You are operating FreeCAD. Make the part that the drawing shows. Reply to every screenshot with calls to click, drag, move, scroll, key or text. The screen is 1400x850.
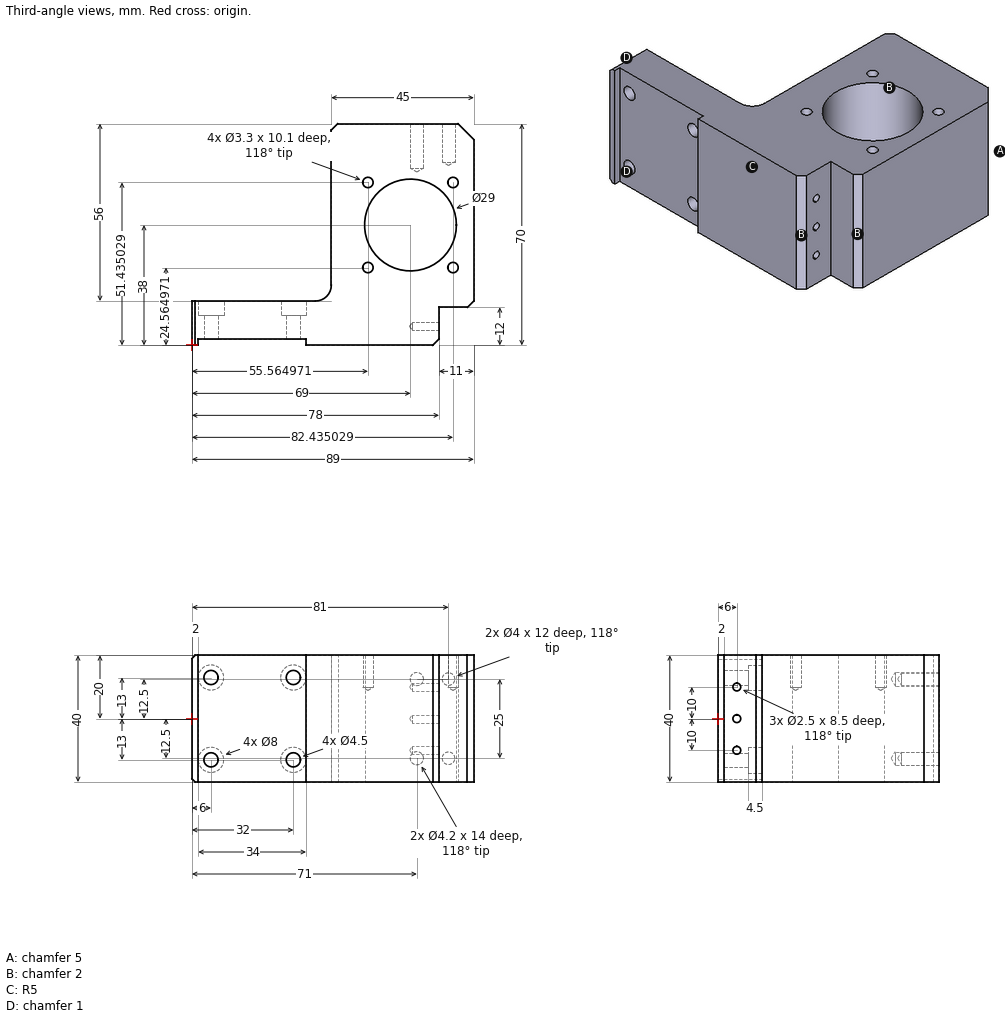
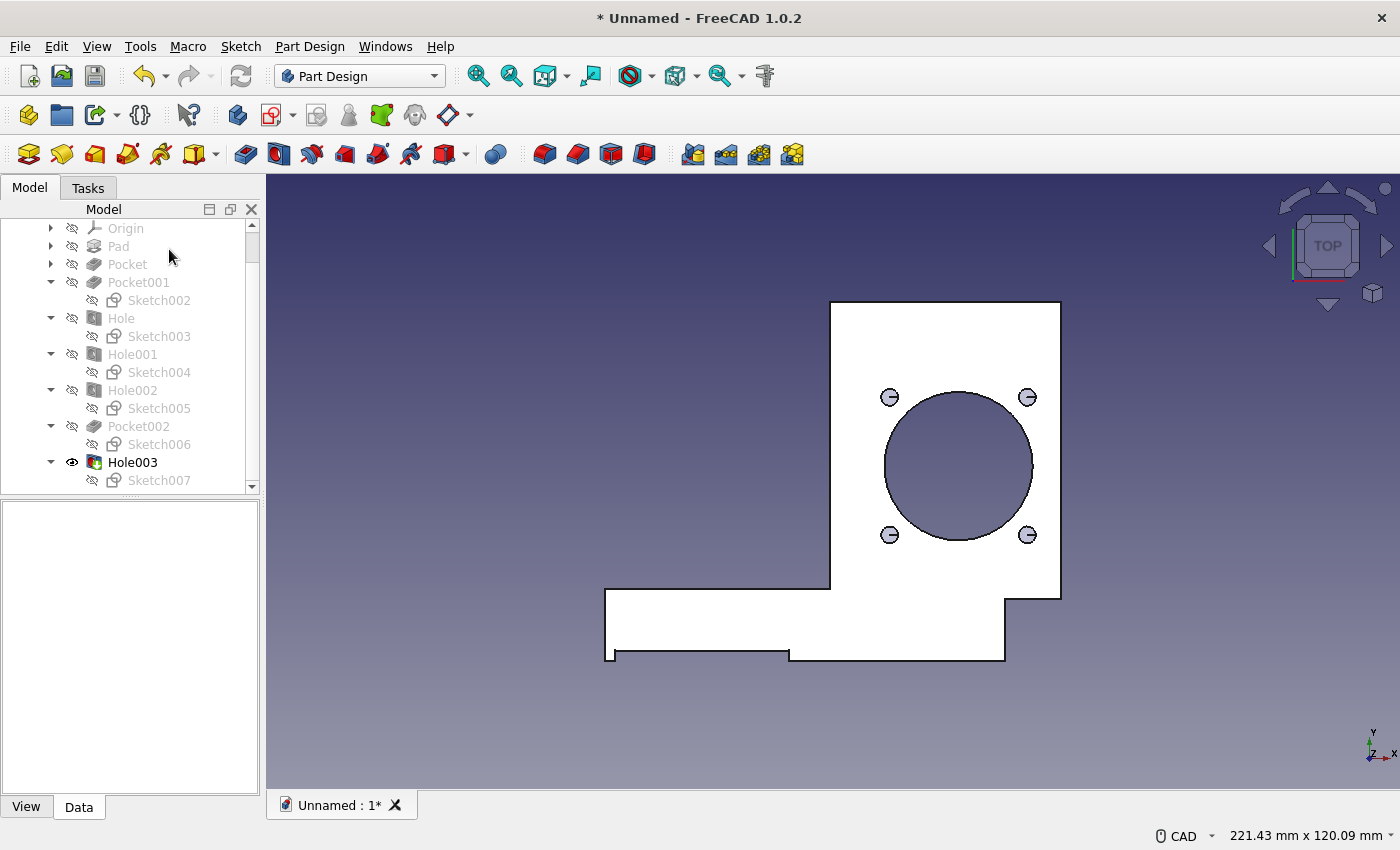
key(0)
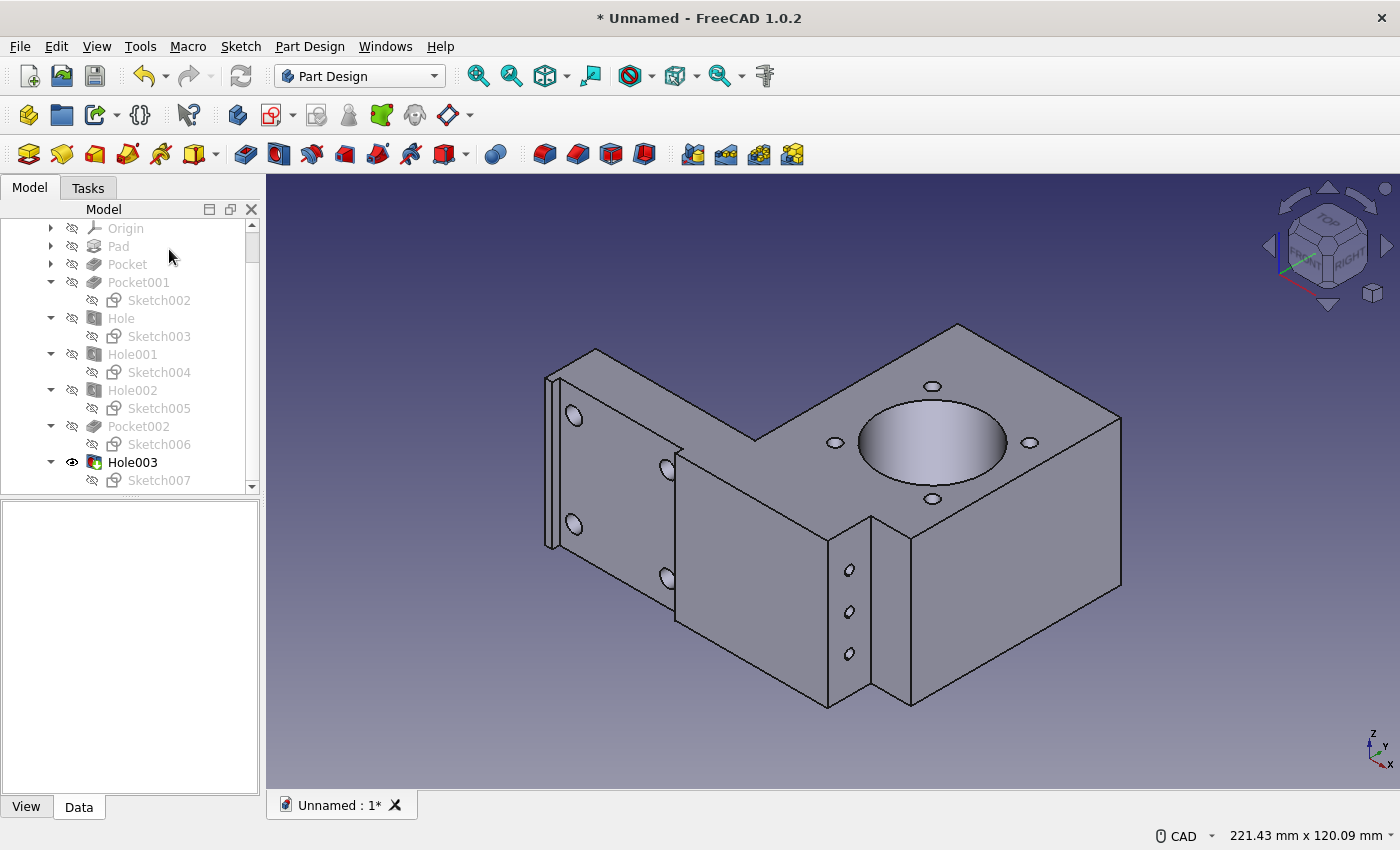
key(1)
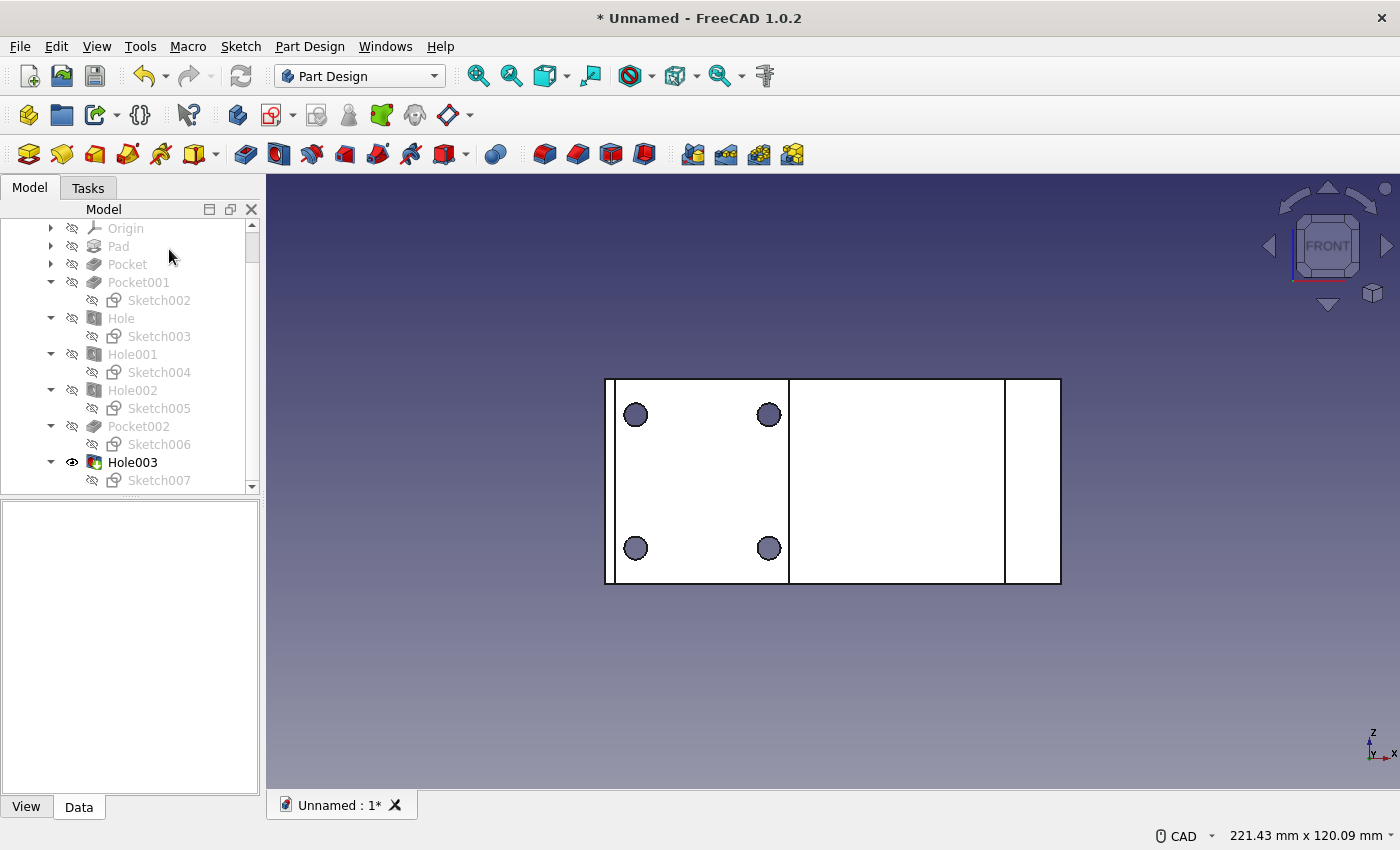
key(v)
key(f)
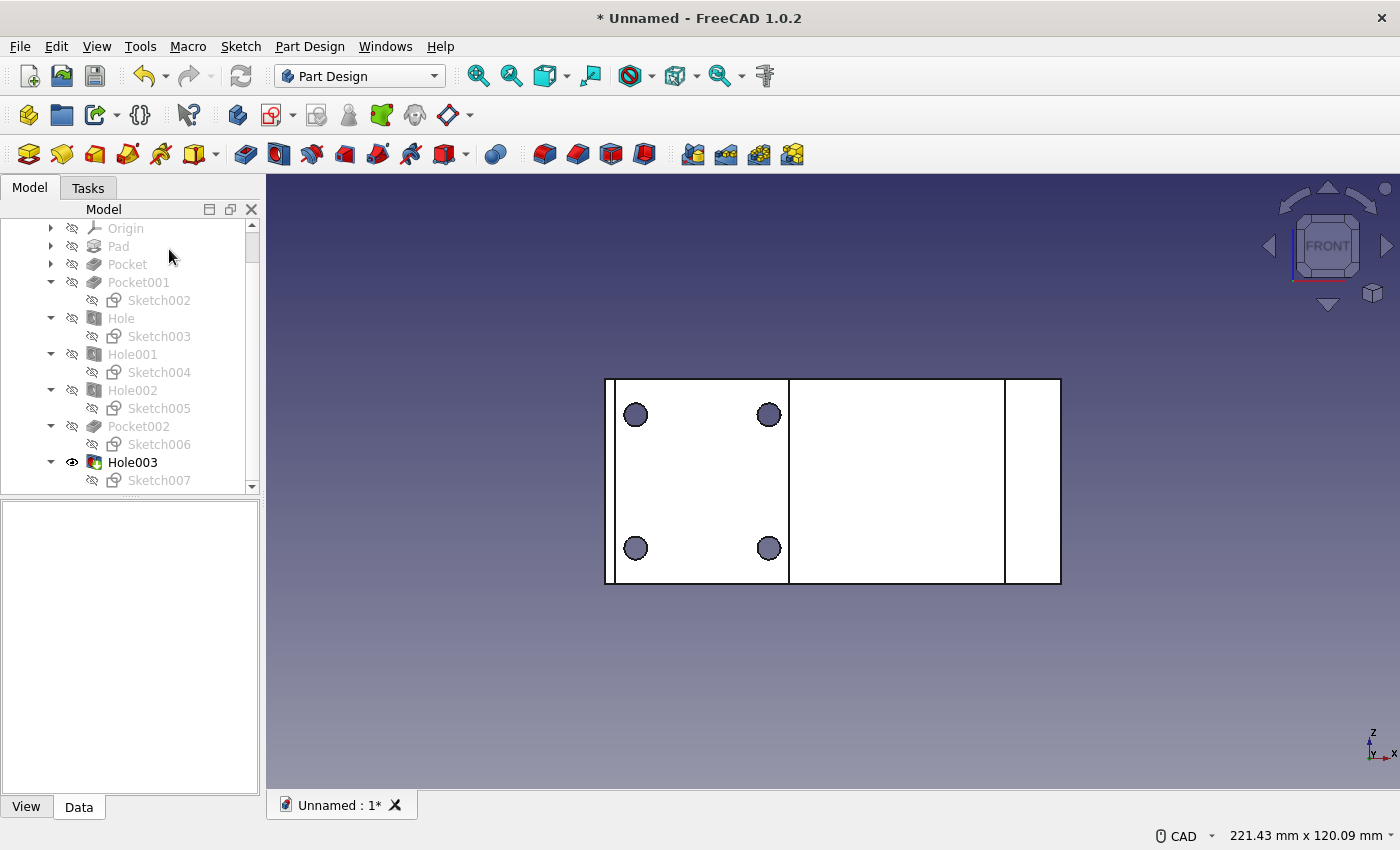
key(3)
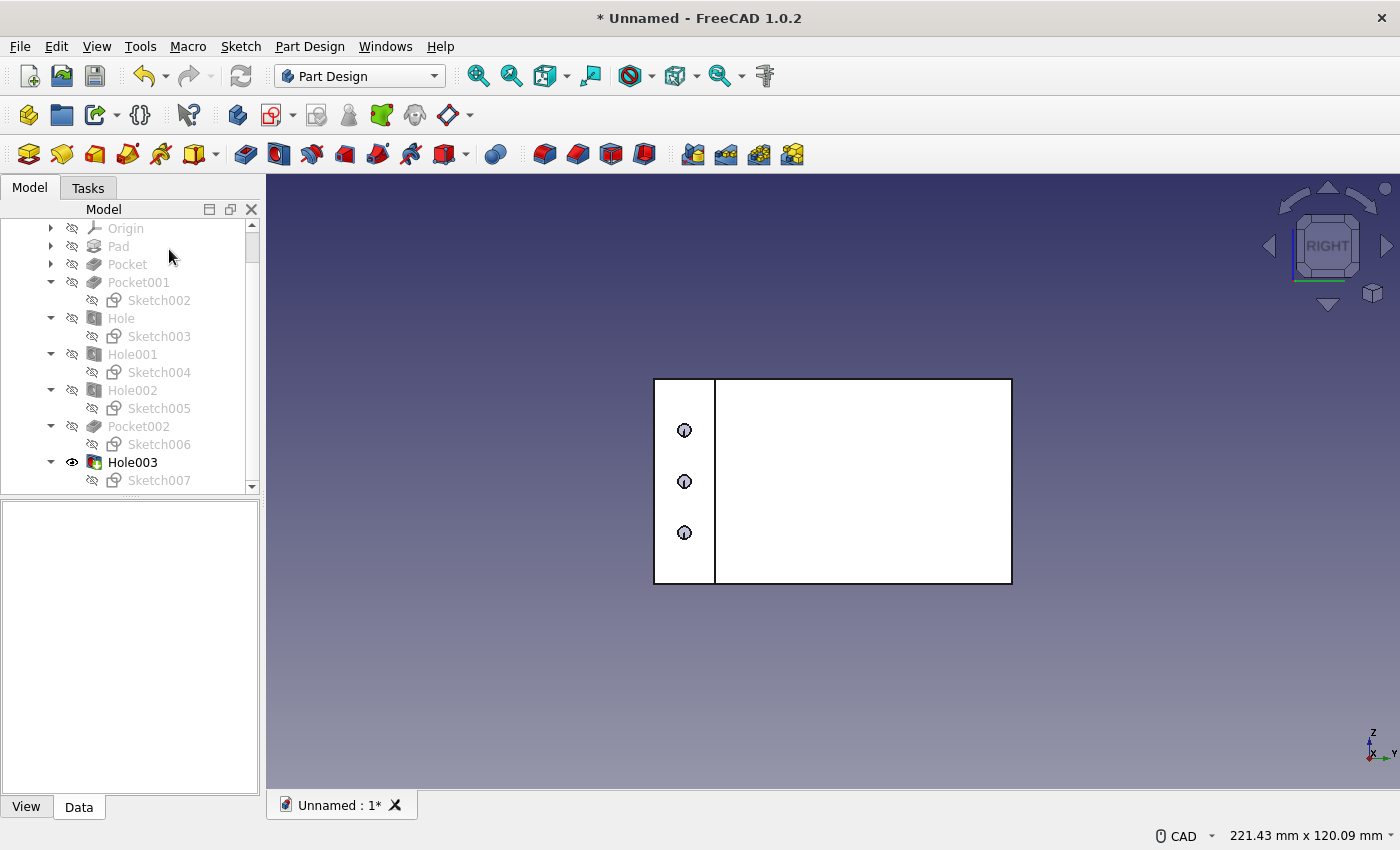
click(479, 76)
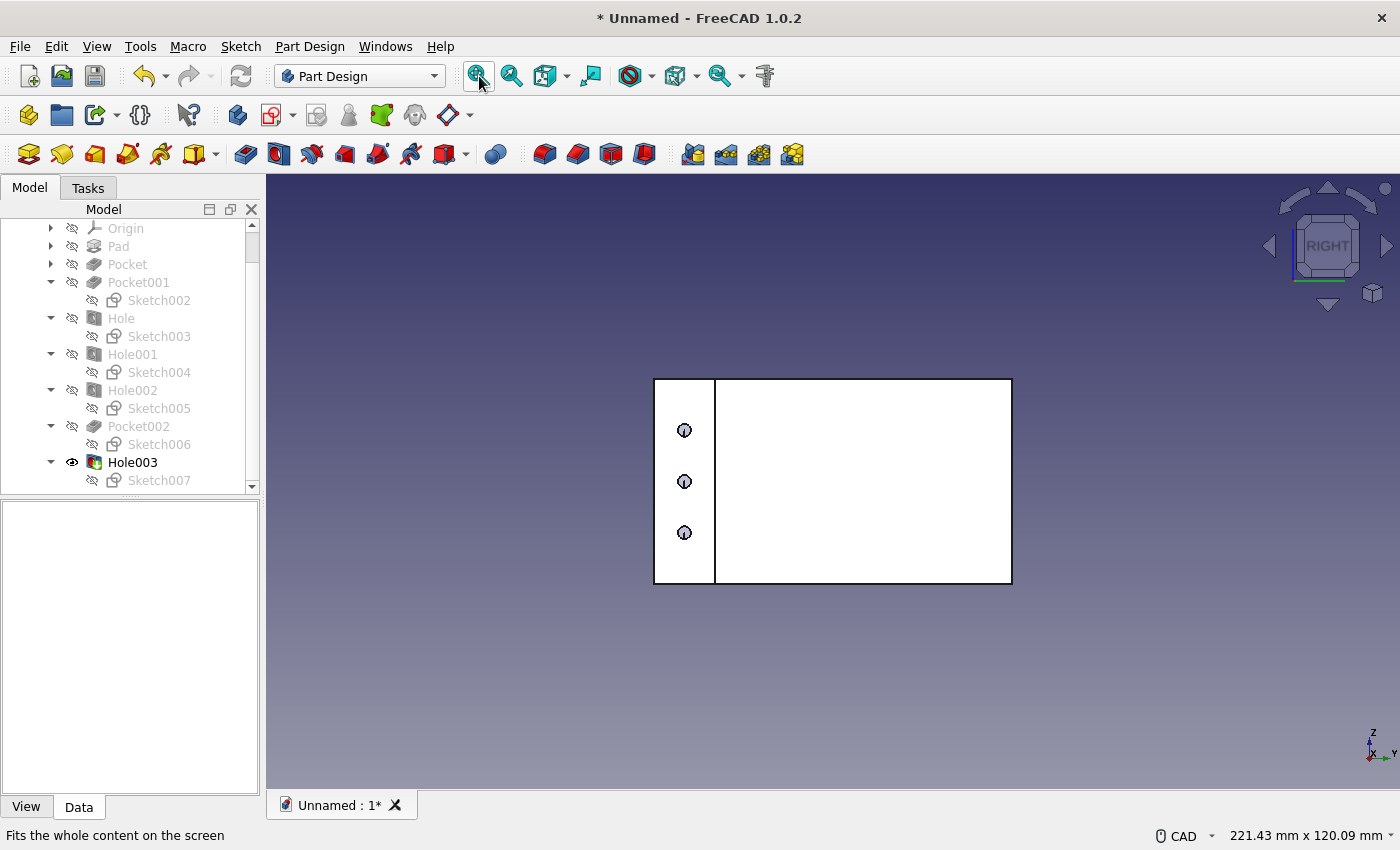
click(1012, 480)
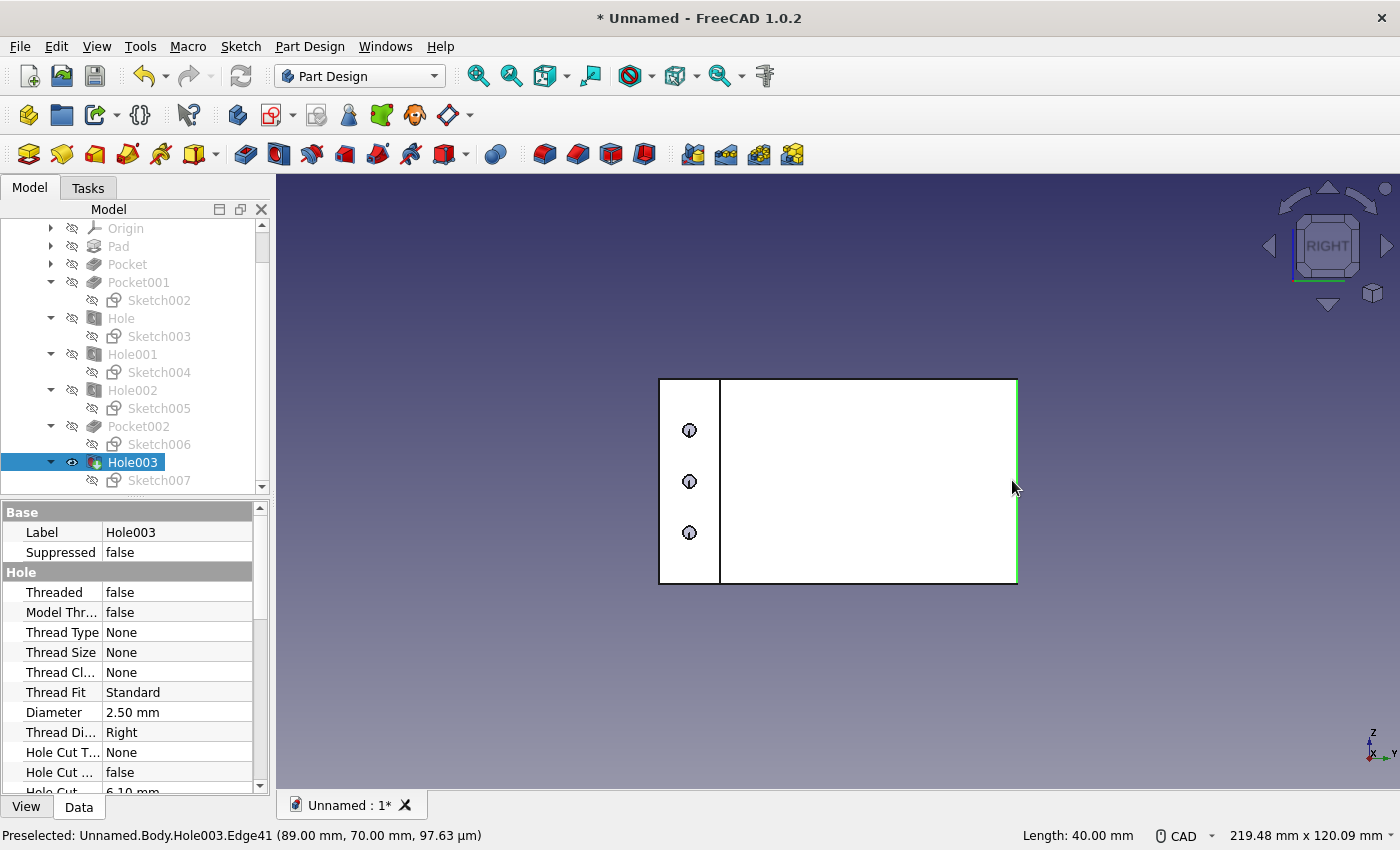
click(578, 154)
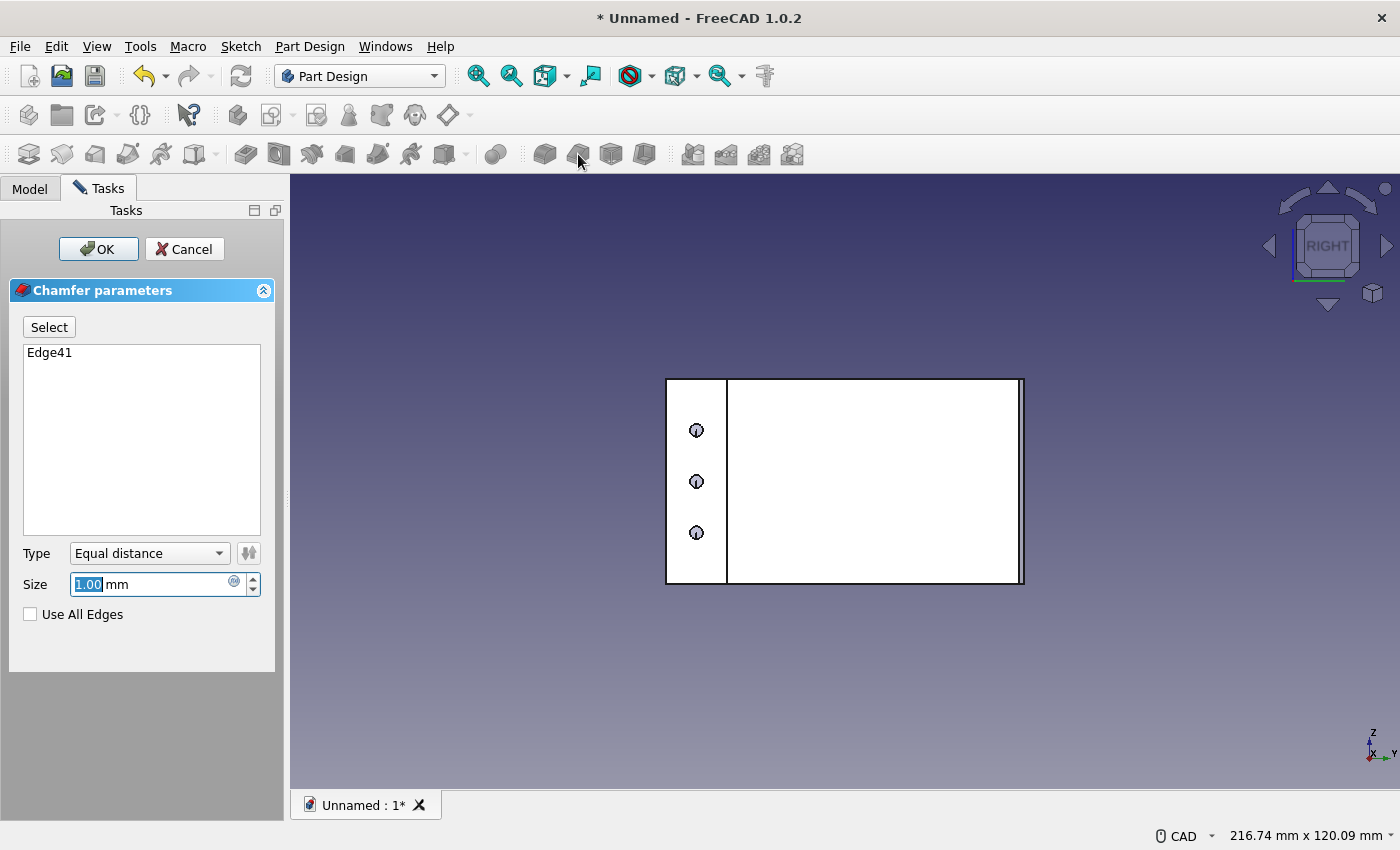
text(5)
key(Tab)